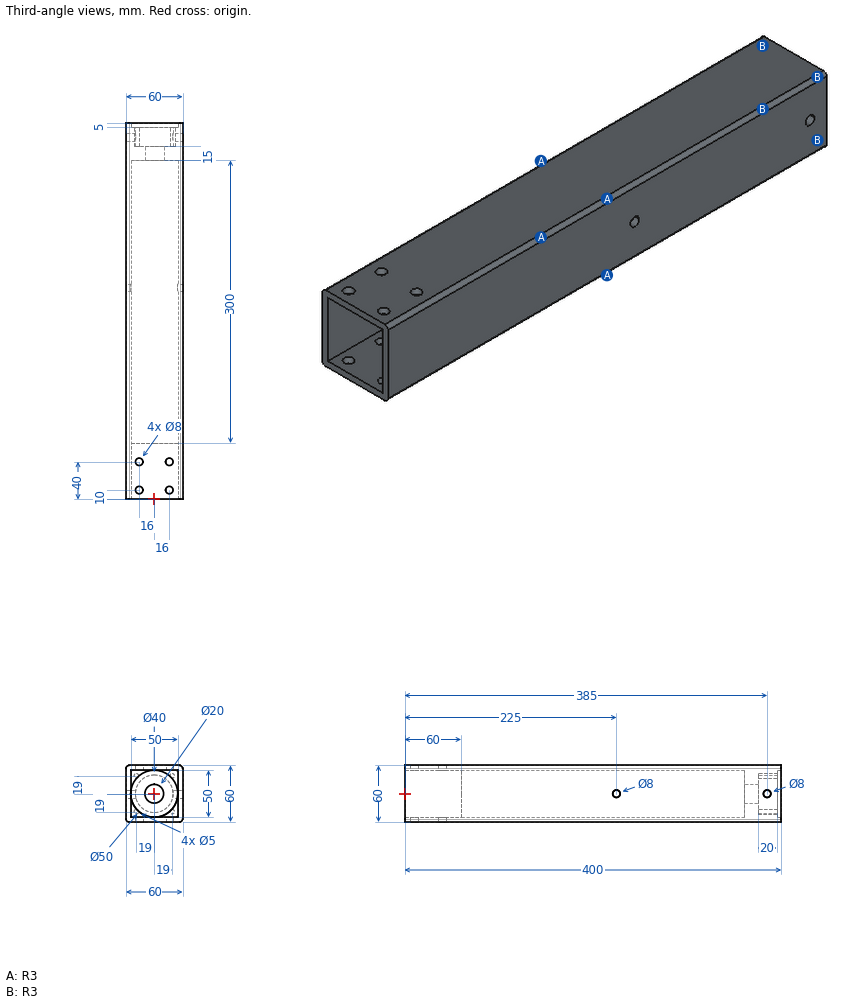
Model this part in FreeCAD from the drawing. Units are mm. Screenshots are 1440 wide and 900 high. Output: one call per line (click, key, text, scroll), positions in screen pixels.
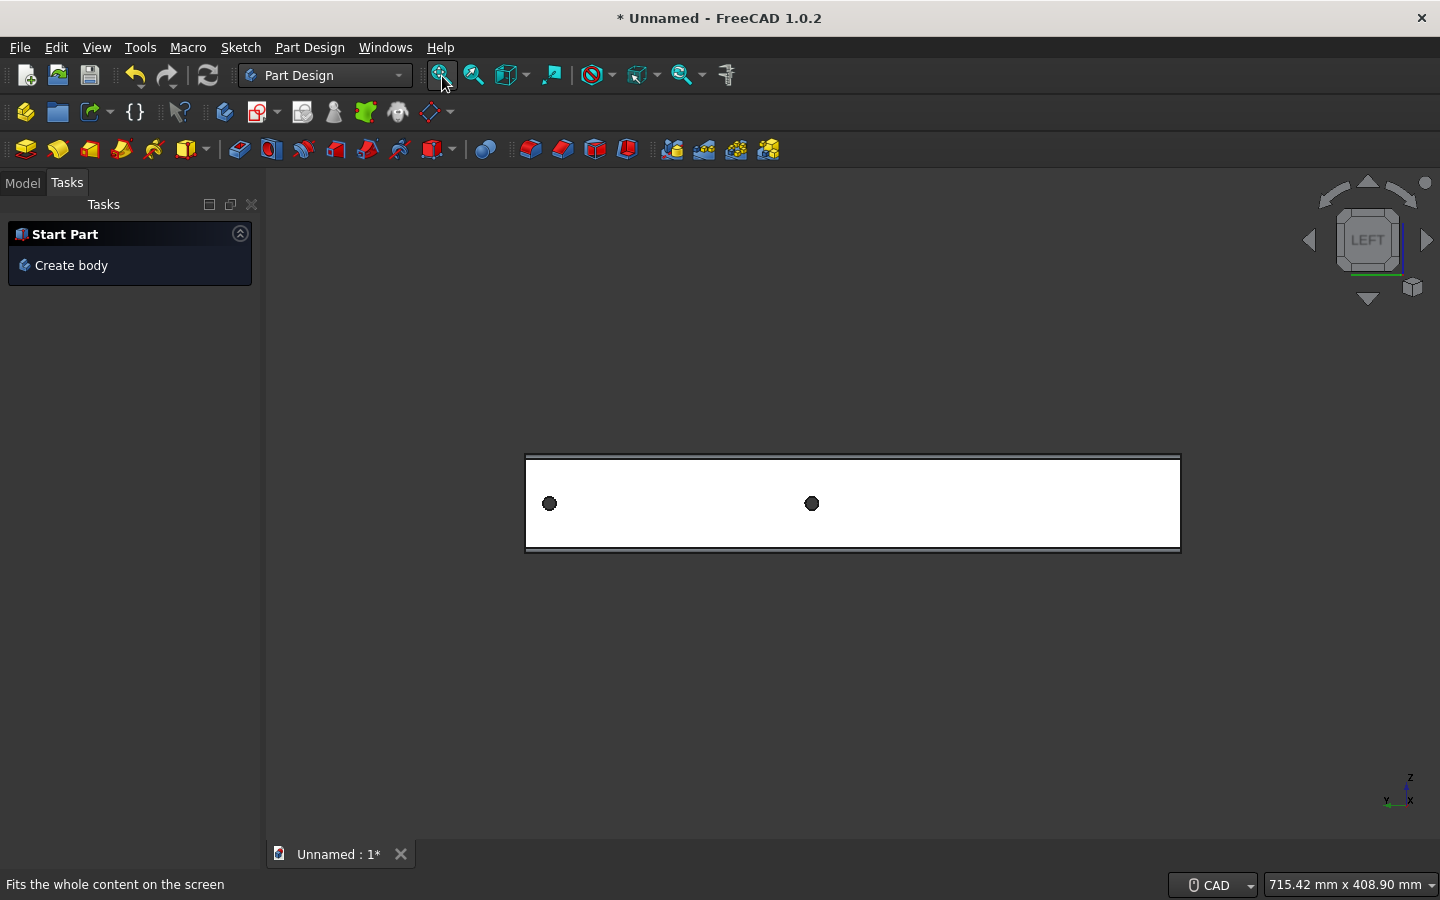
key(v)
key(3)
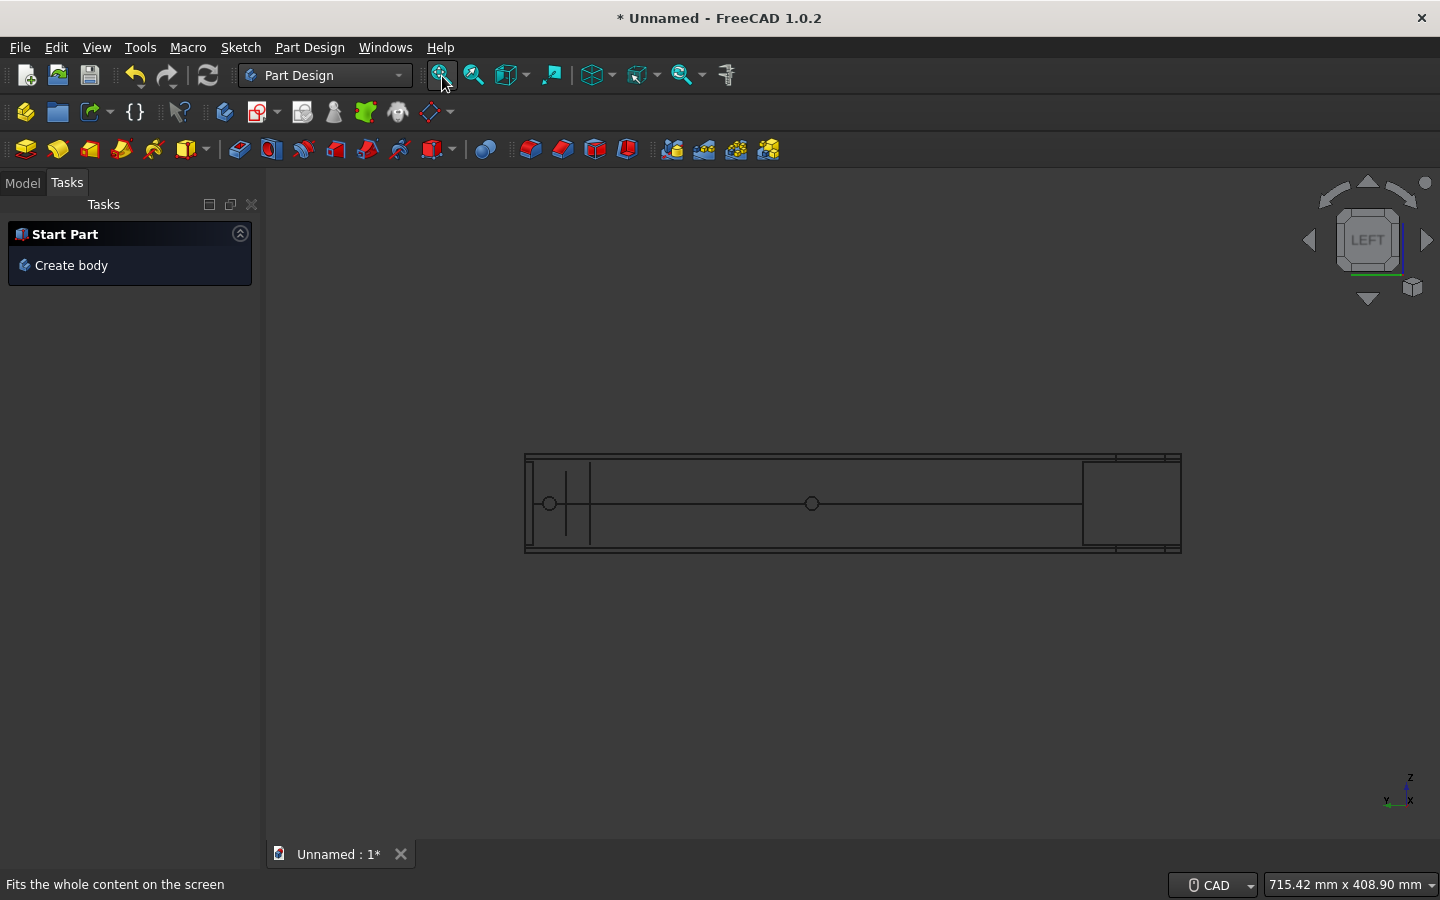
key(0)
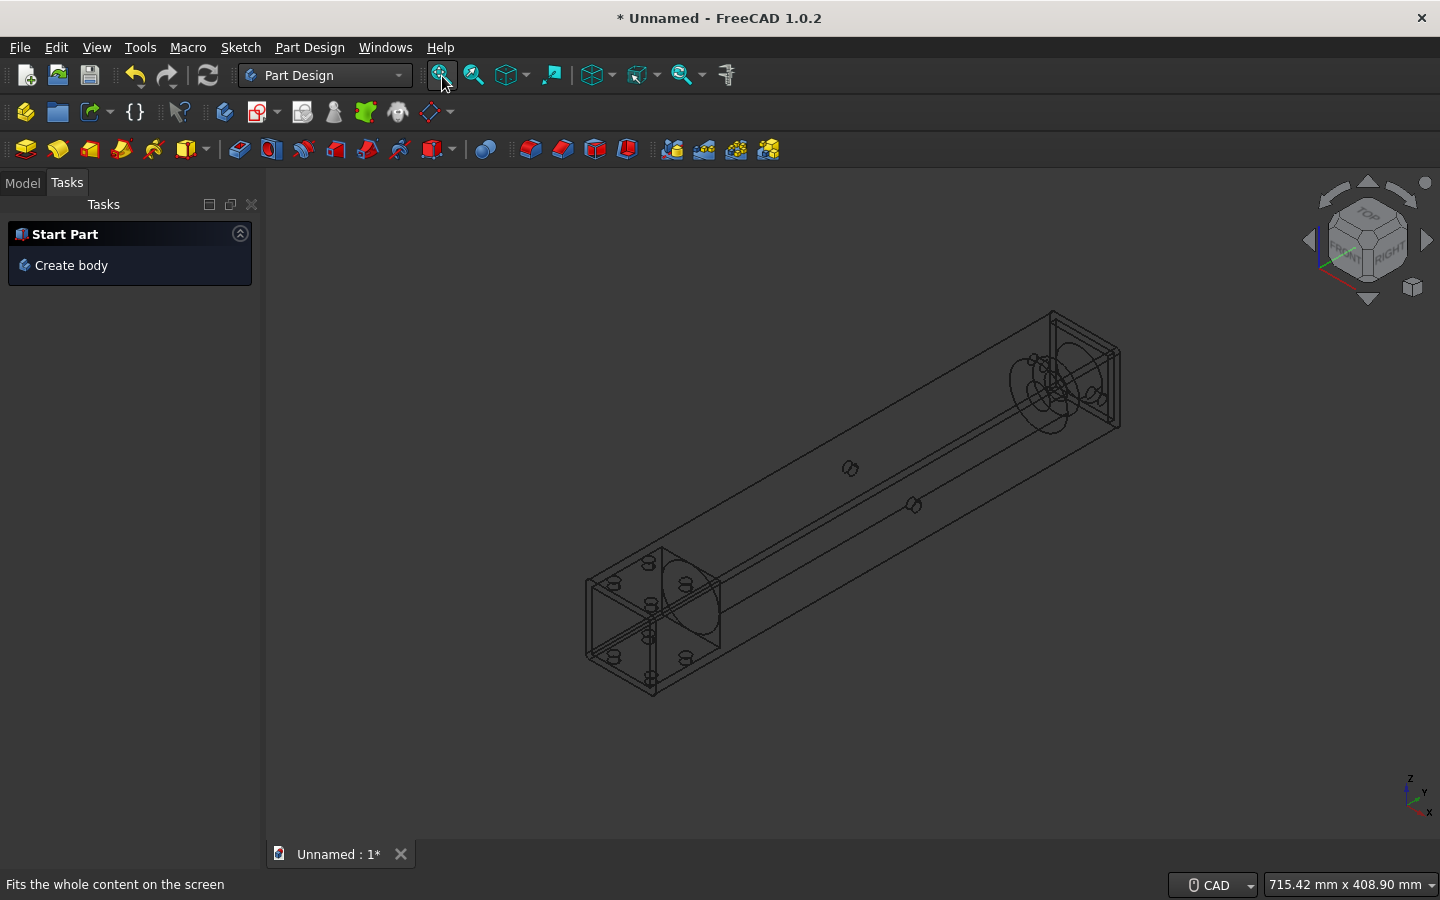
scroll(1111, 420, up, 8)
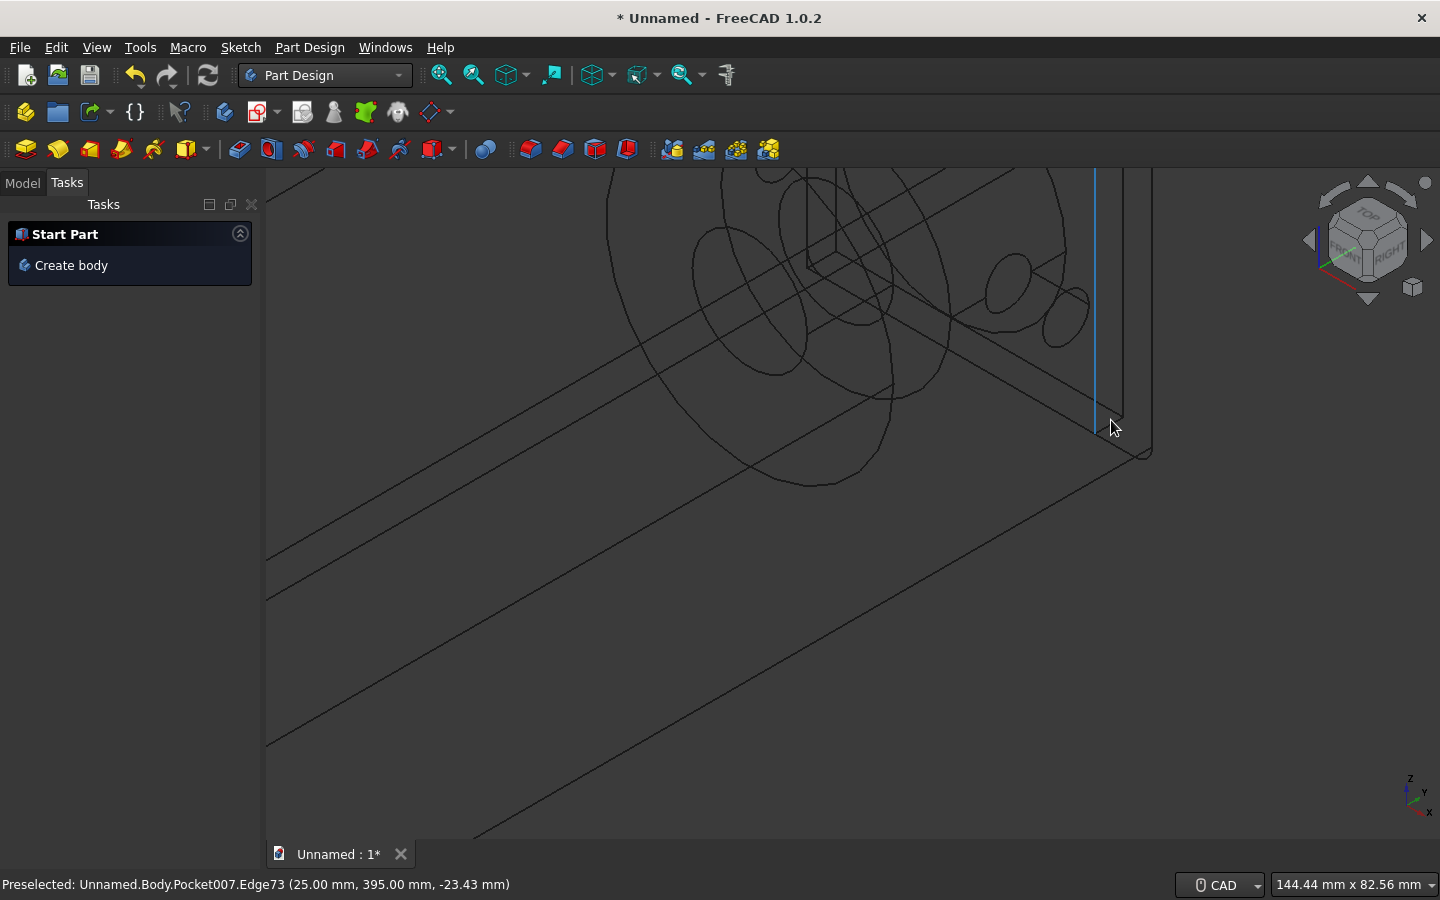
click(1109, 425)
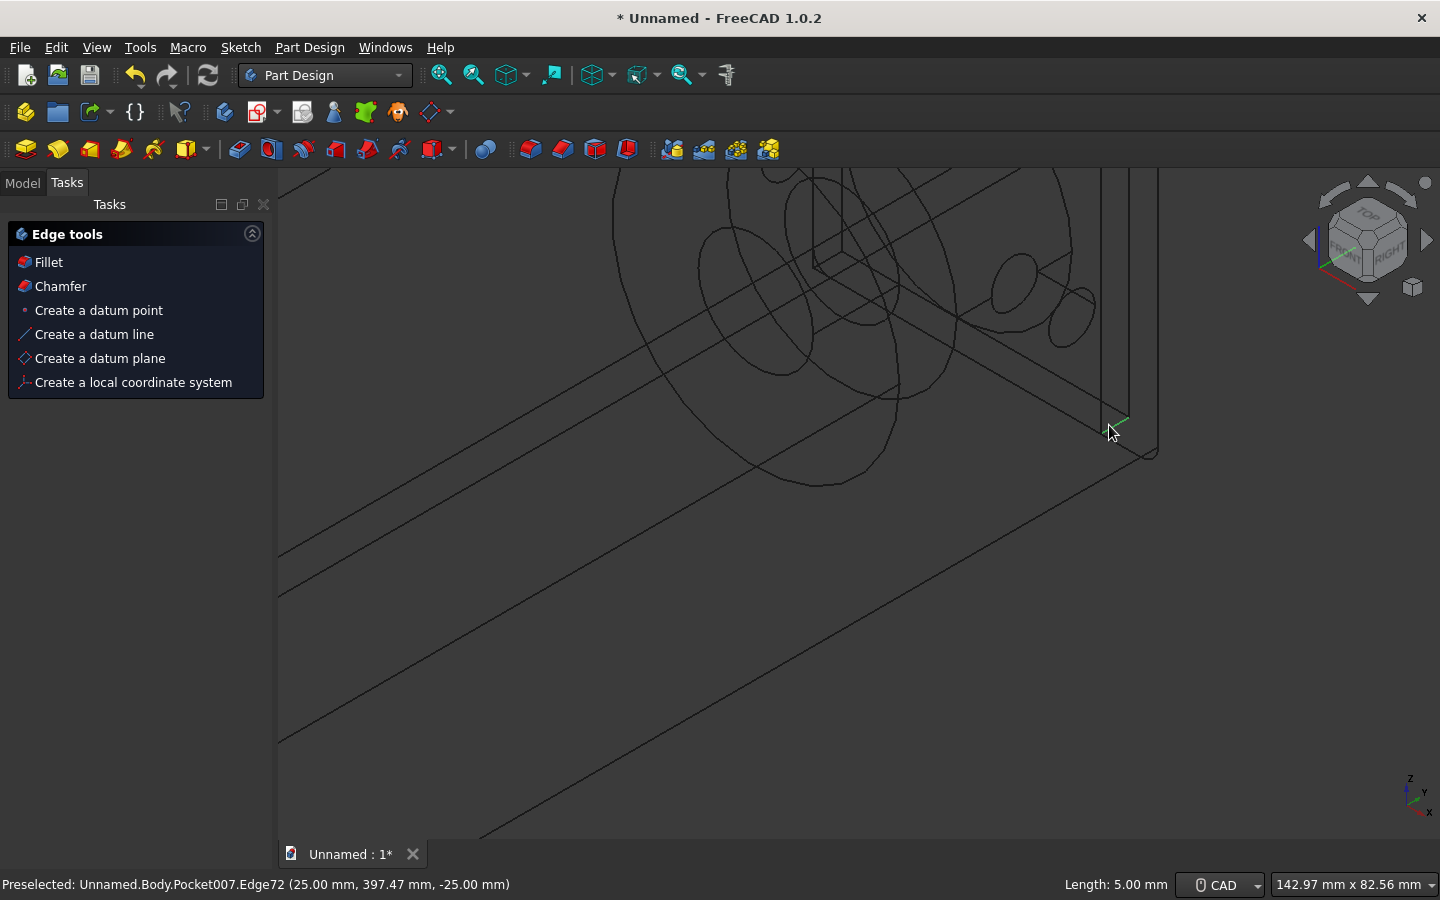
click(828, 259, ctrl)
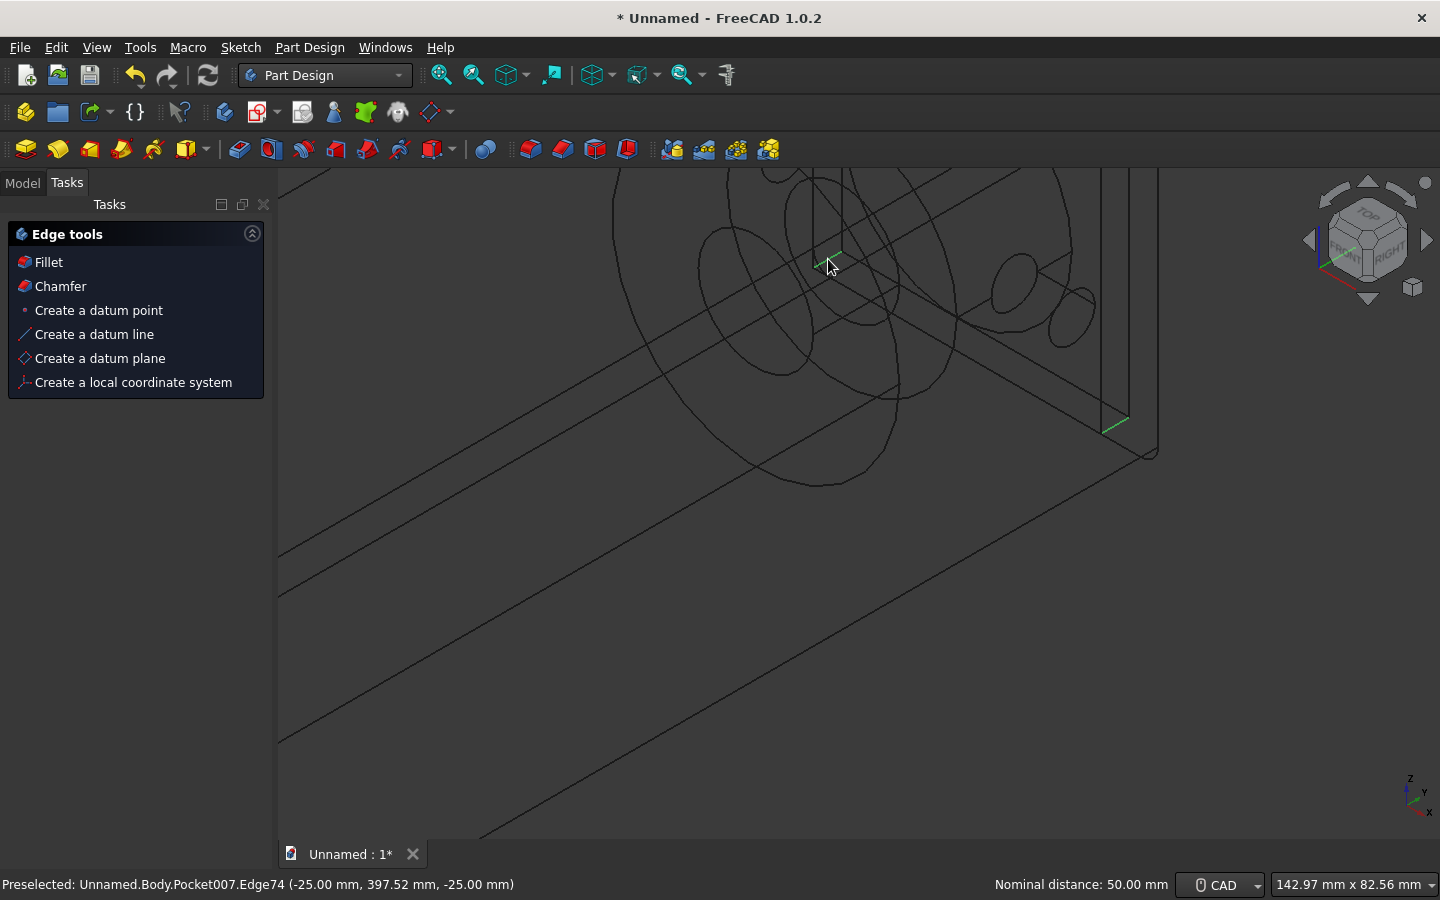
click(442, 76)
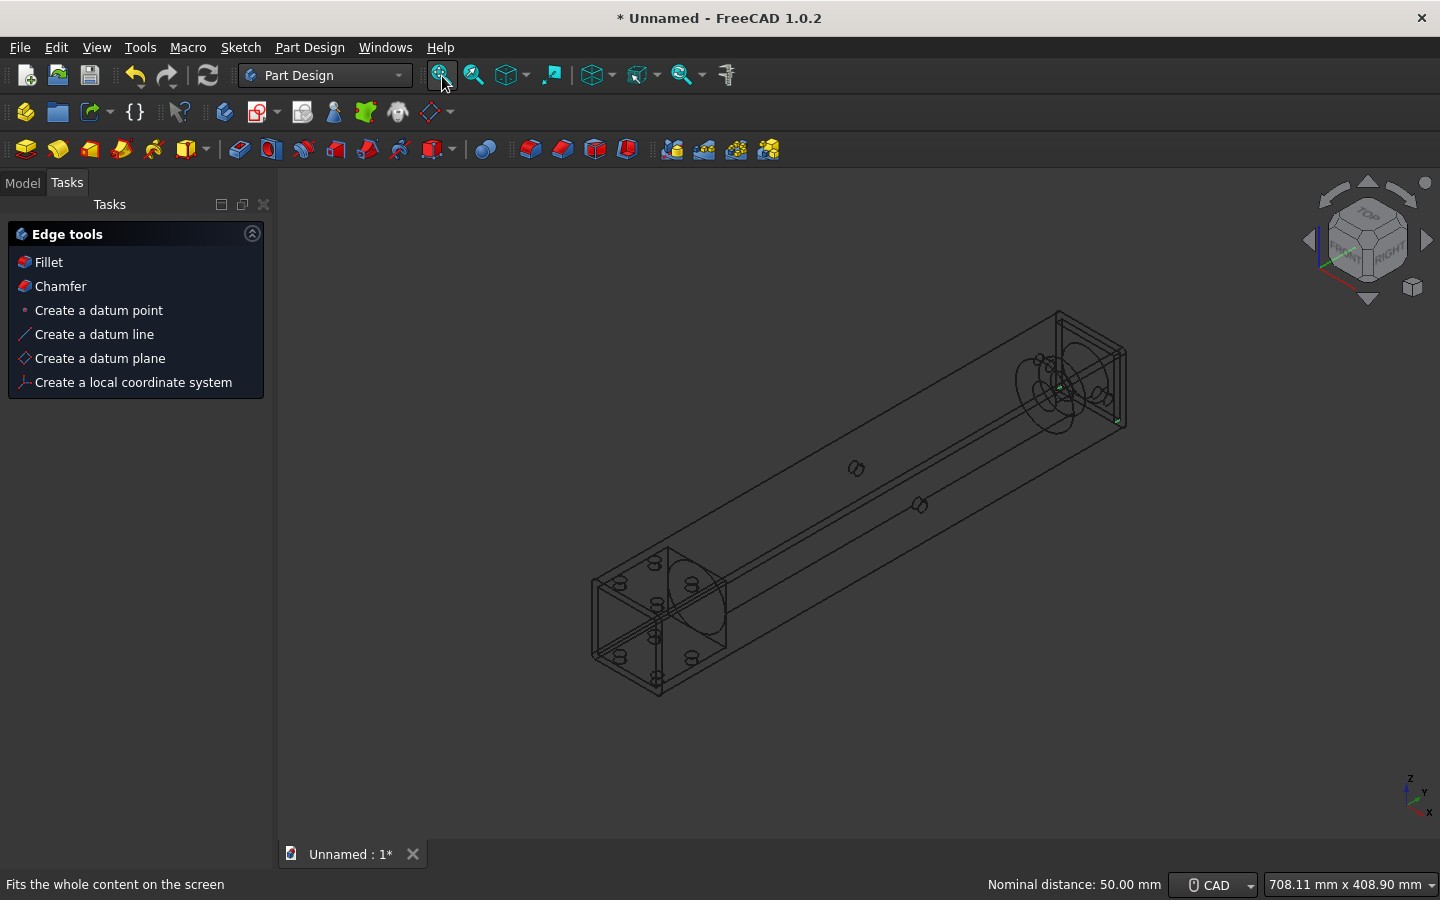
key(2)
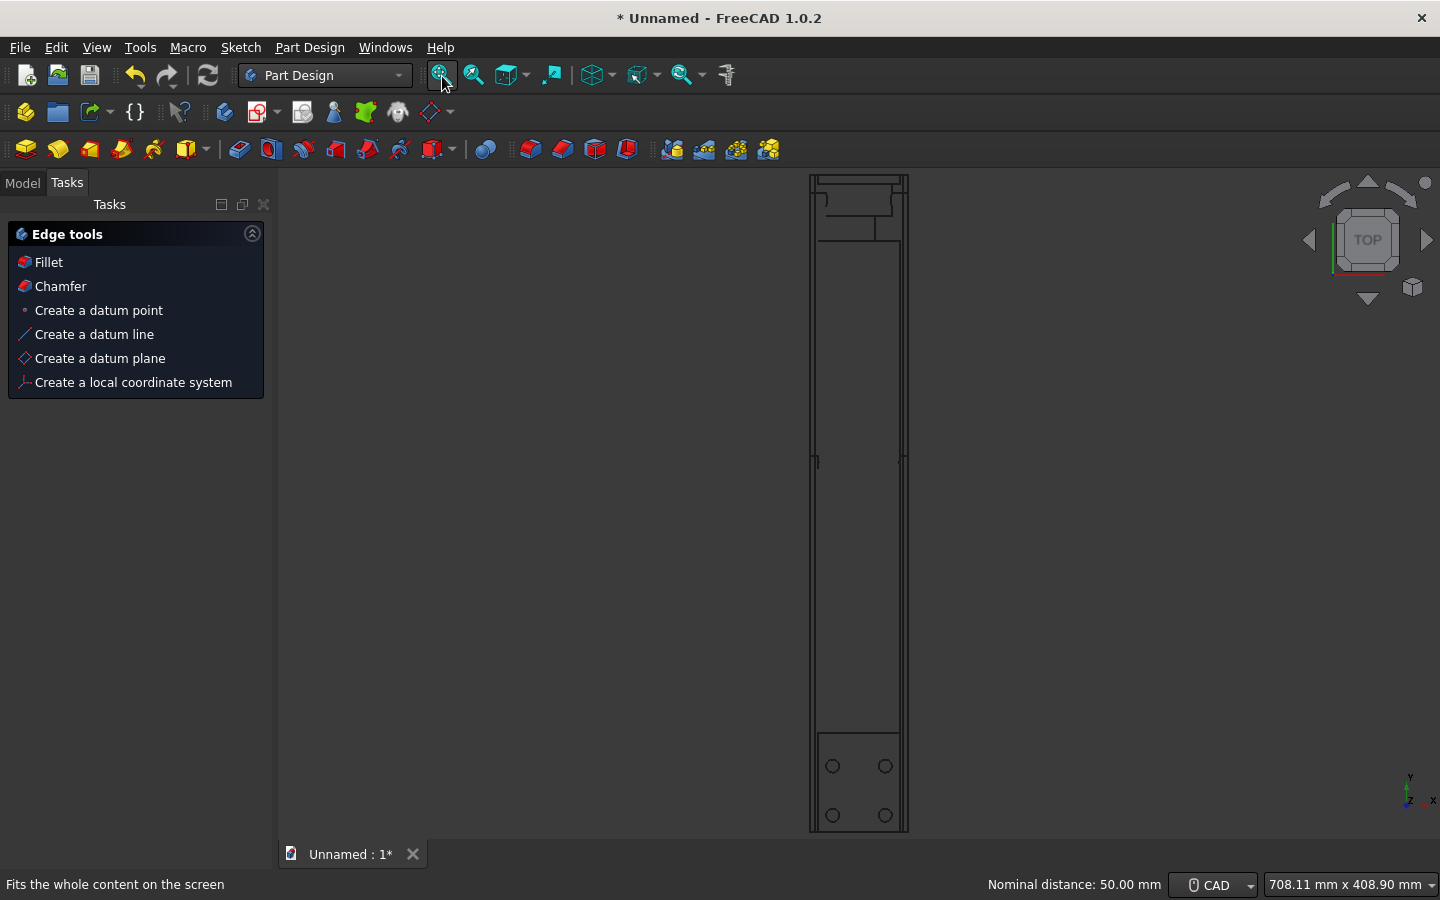
key(1)